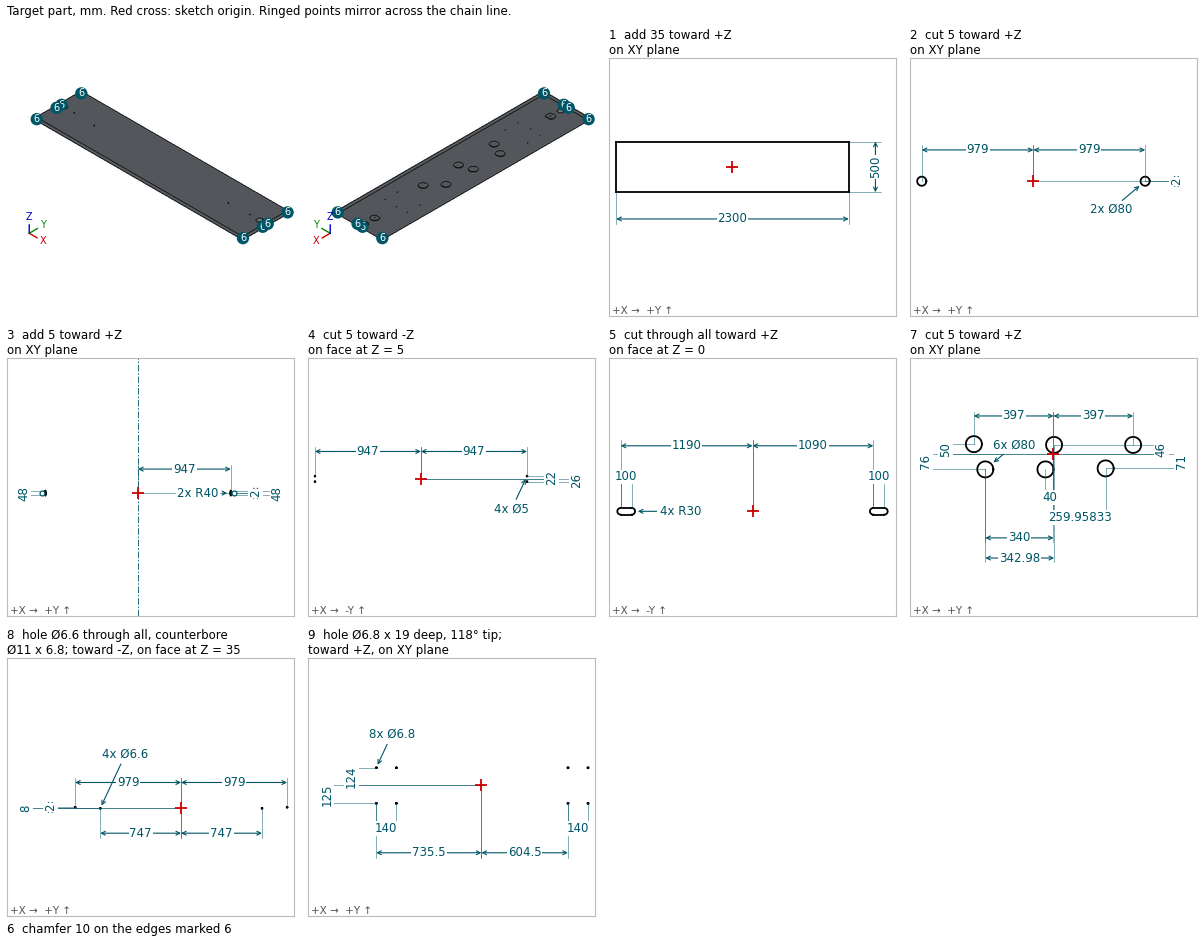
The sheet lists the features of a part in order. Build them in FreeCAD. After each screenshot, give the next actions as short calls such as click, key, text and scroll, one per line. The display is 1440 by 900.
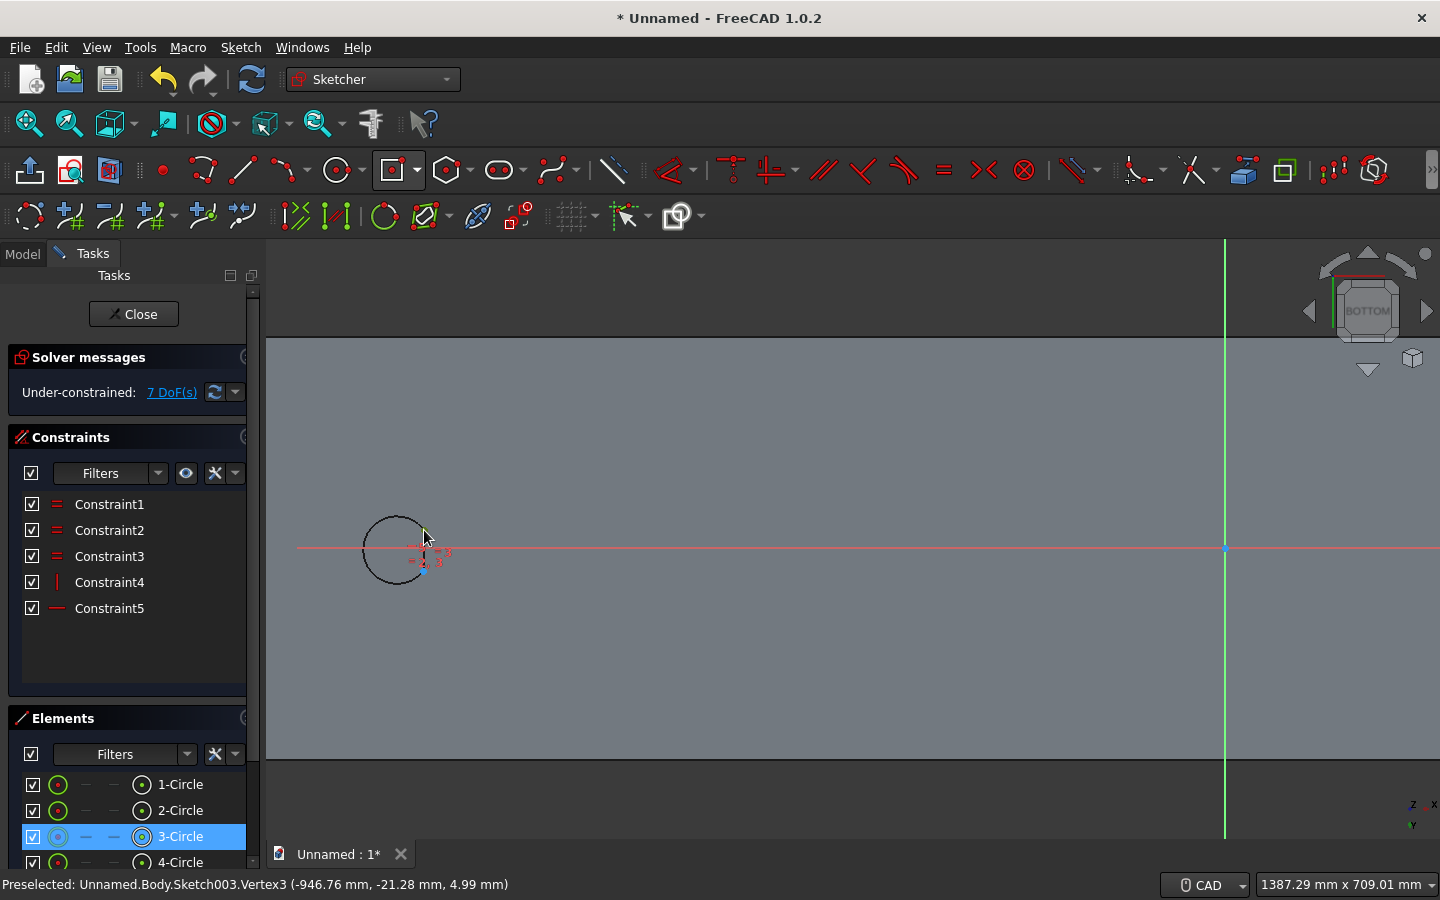
click(424, 571)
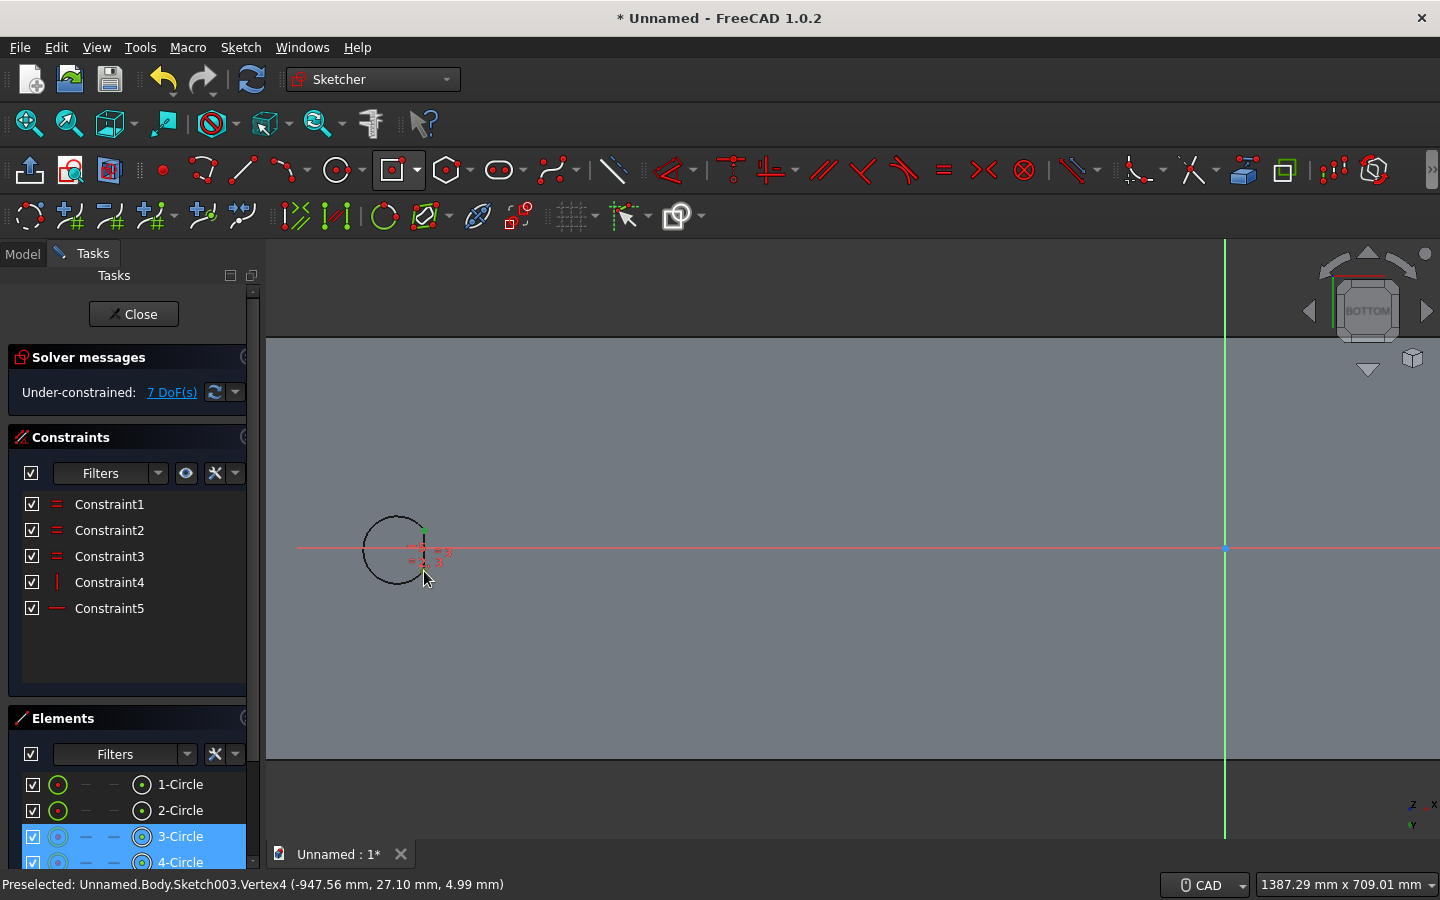
key(v)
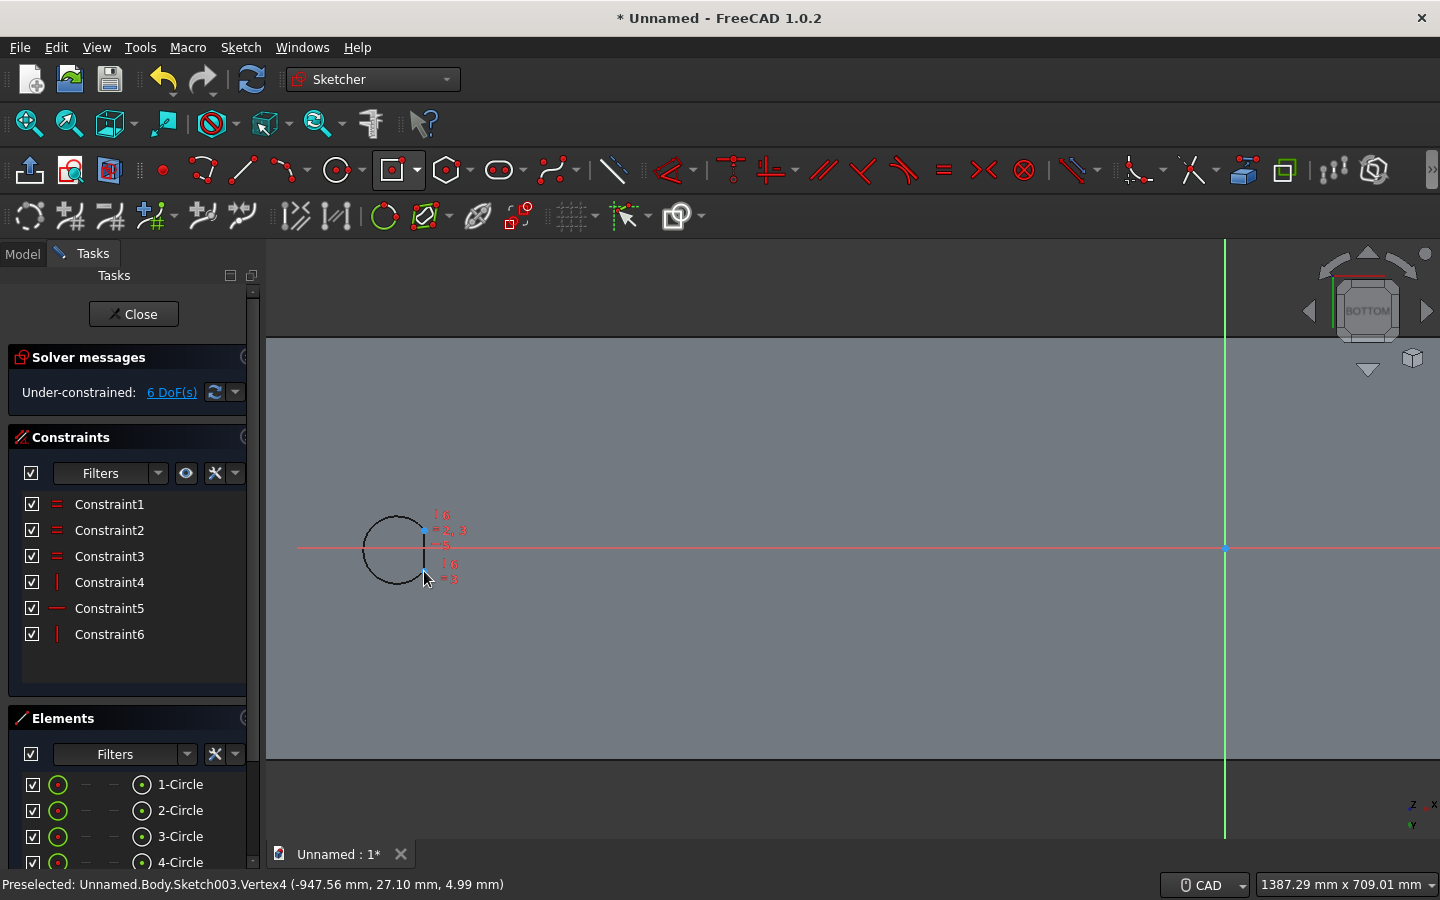
scroll(425, 530, down, 4)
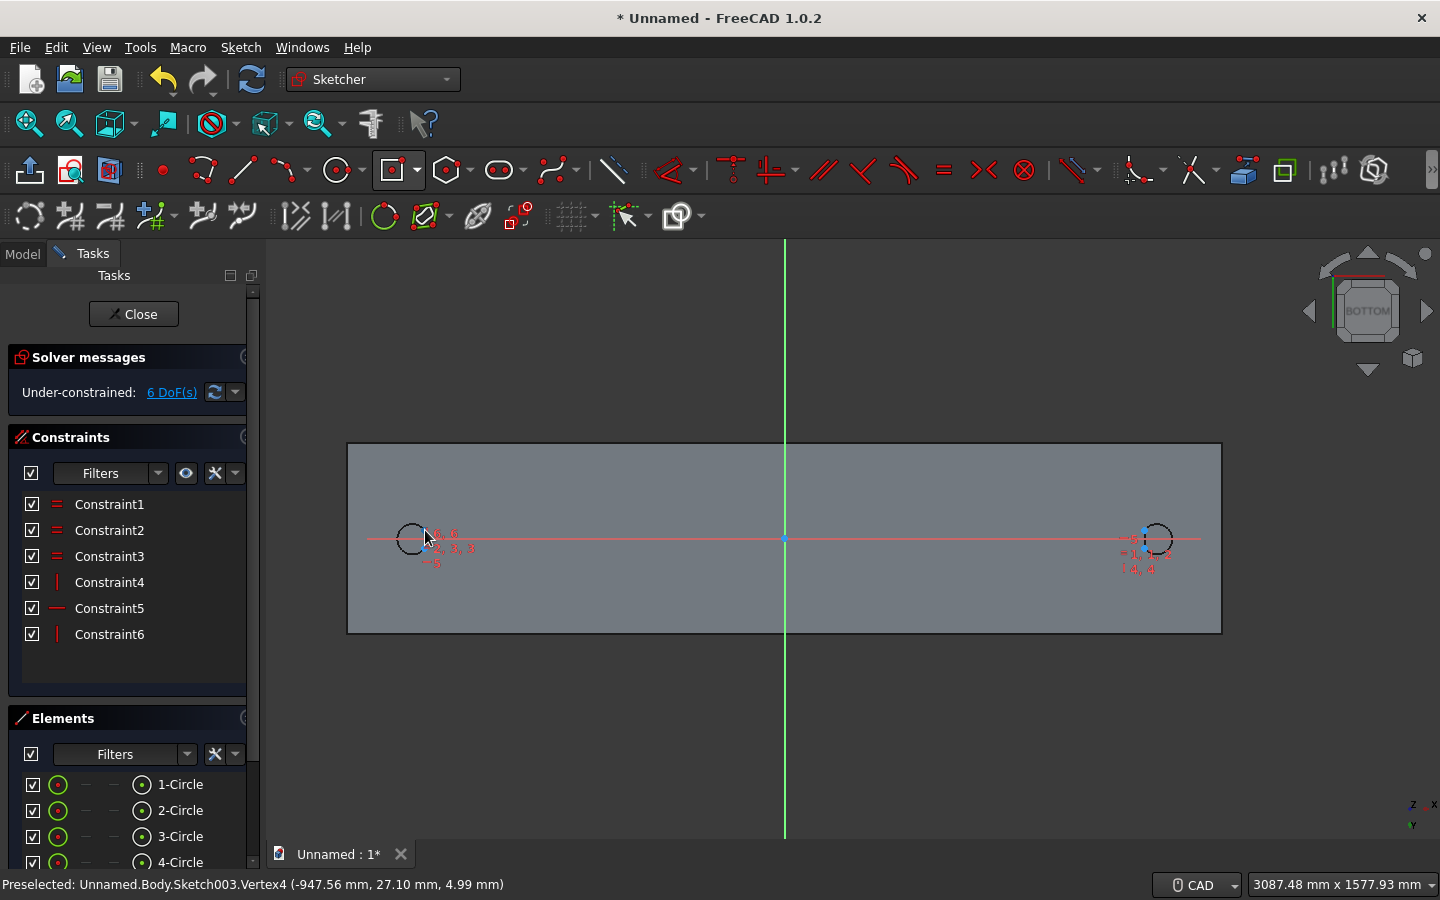
click(1145, 549)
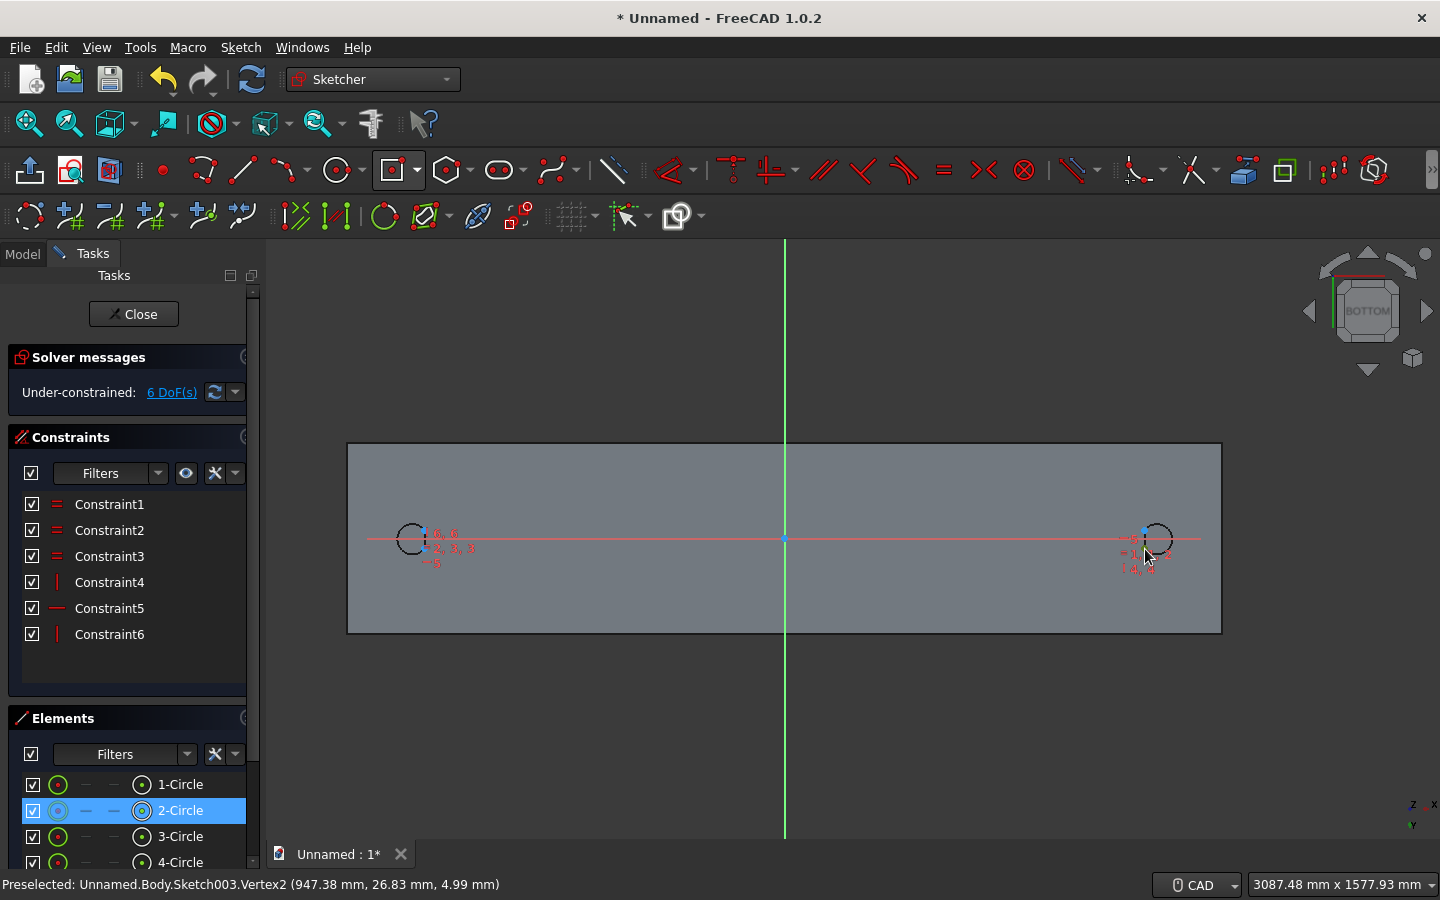
scroll(425, 549, up, 4)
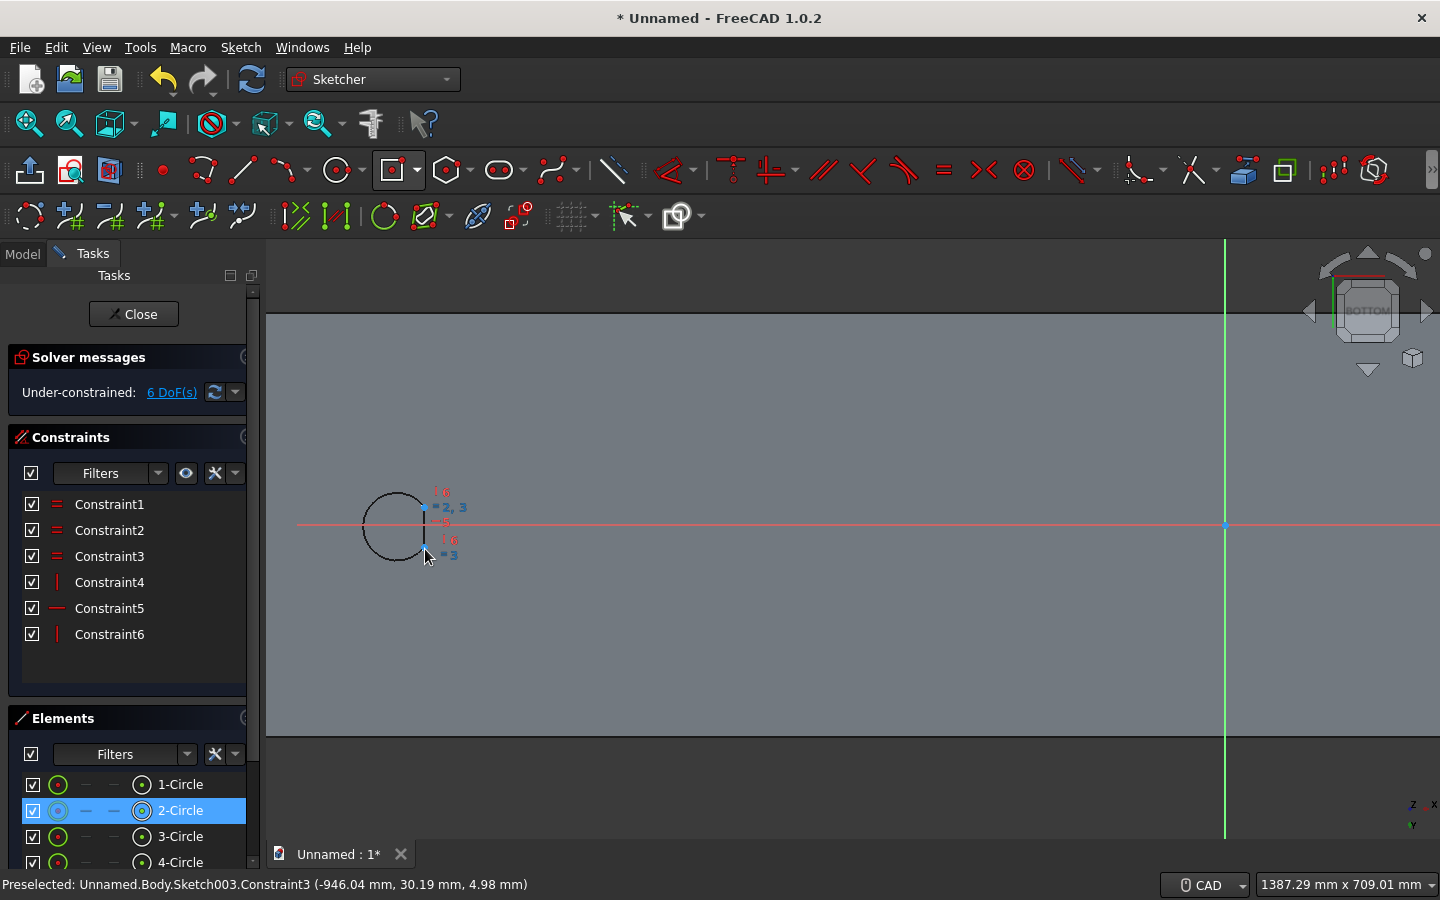
click(424, 548)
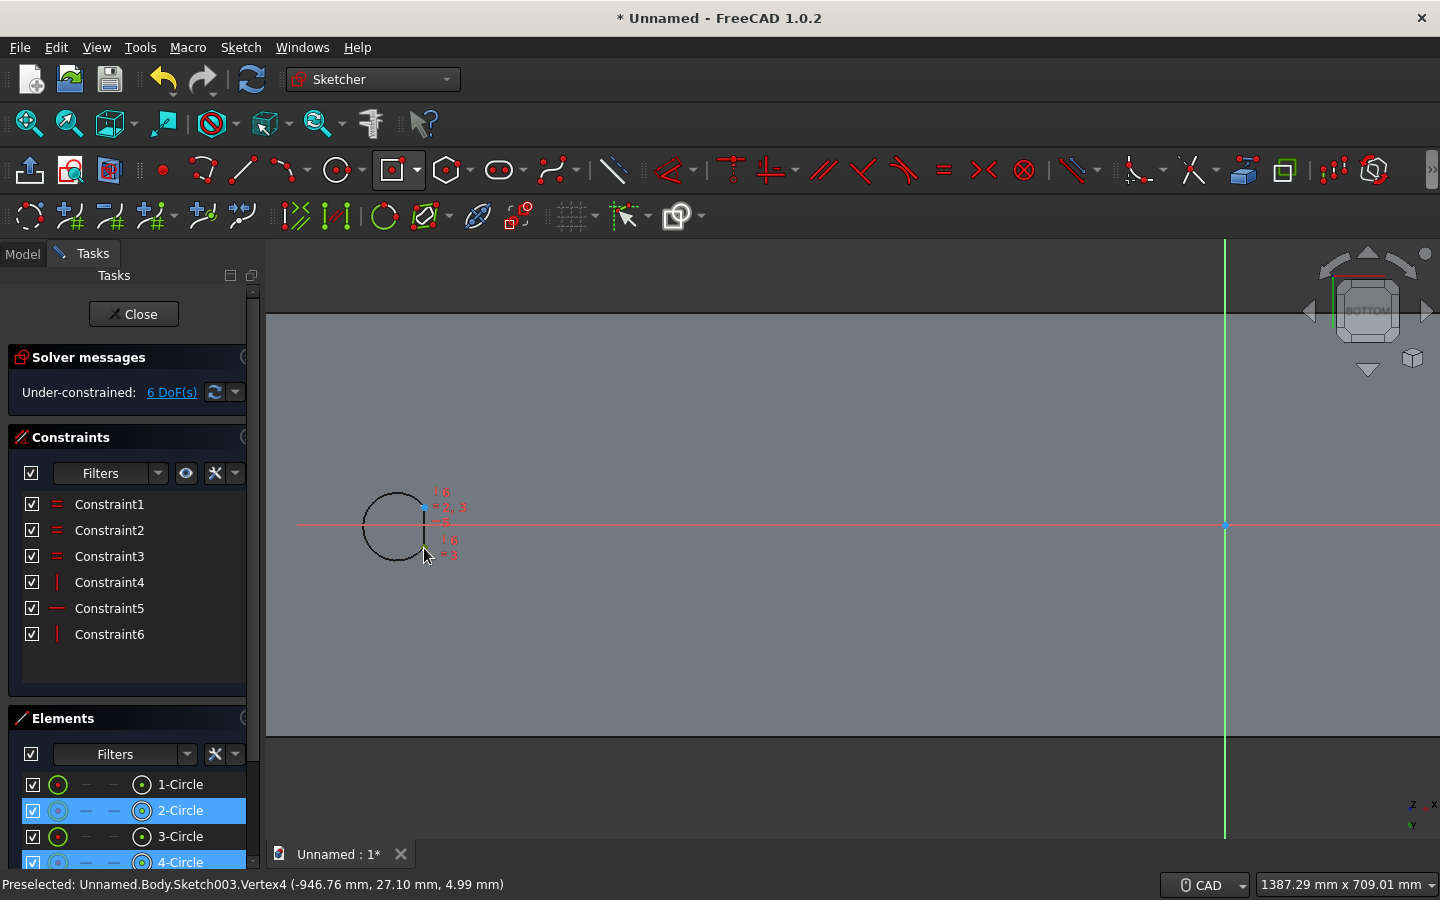
key(h)